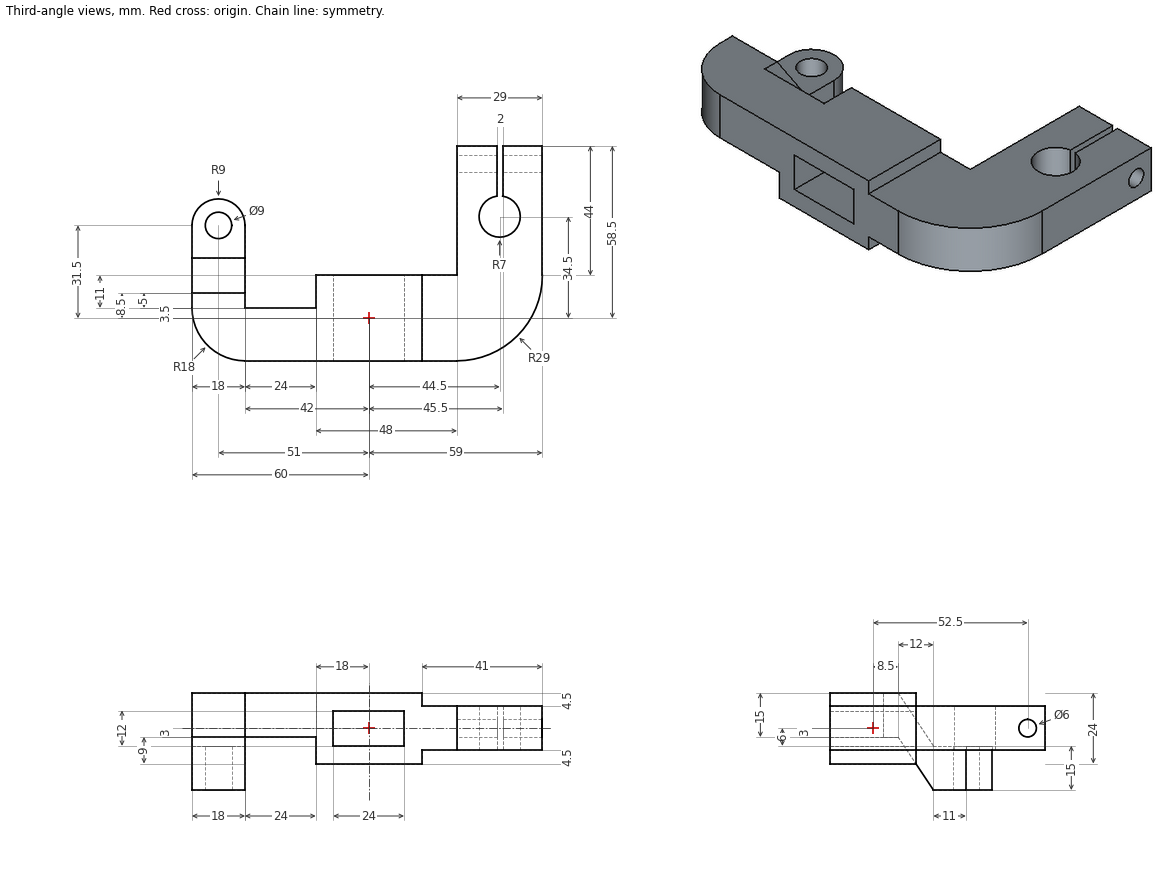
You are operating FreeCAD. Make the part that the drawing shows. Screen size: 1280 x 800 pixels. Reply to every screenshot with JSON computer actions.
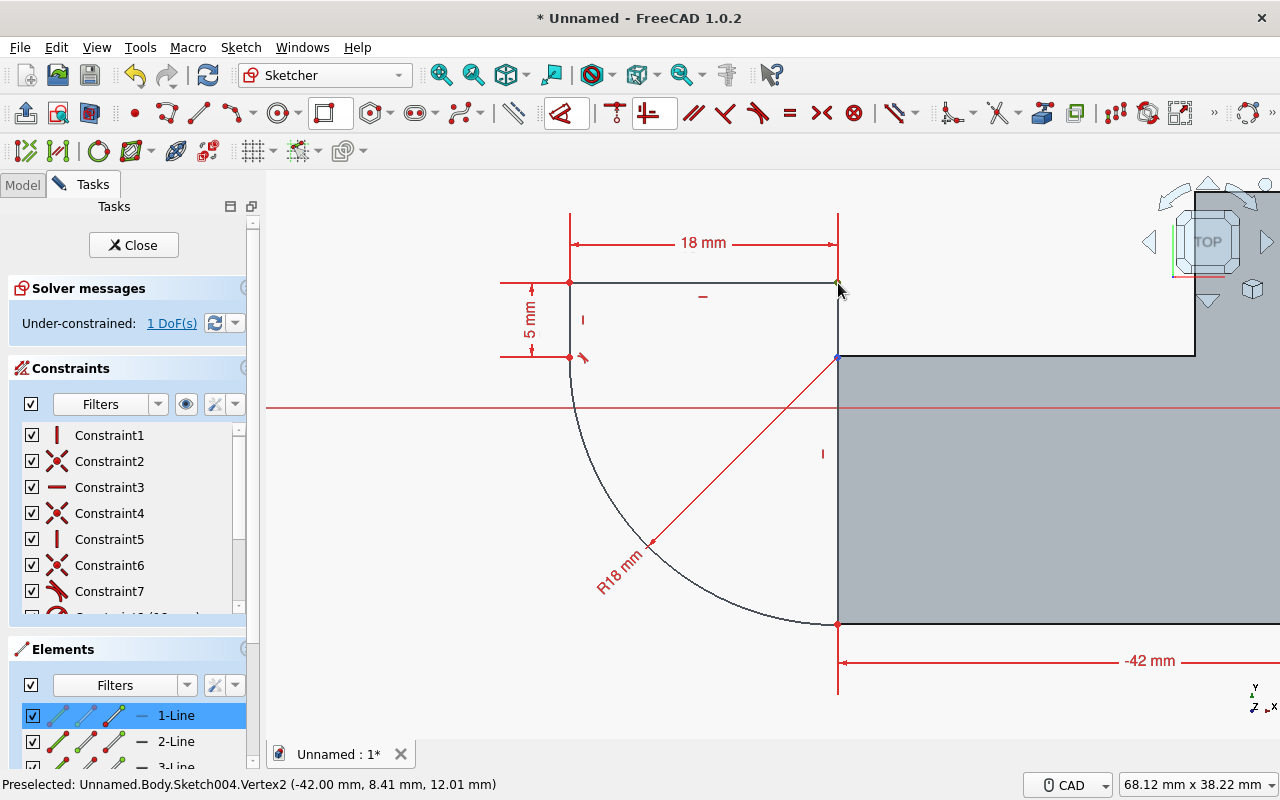
{"action": "key", "text": "i"}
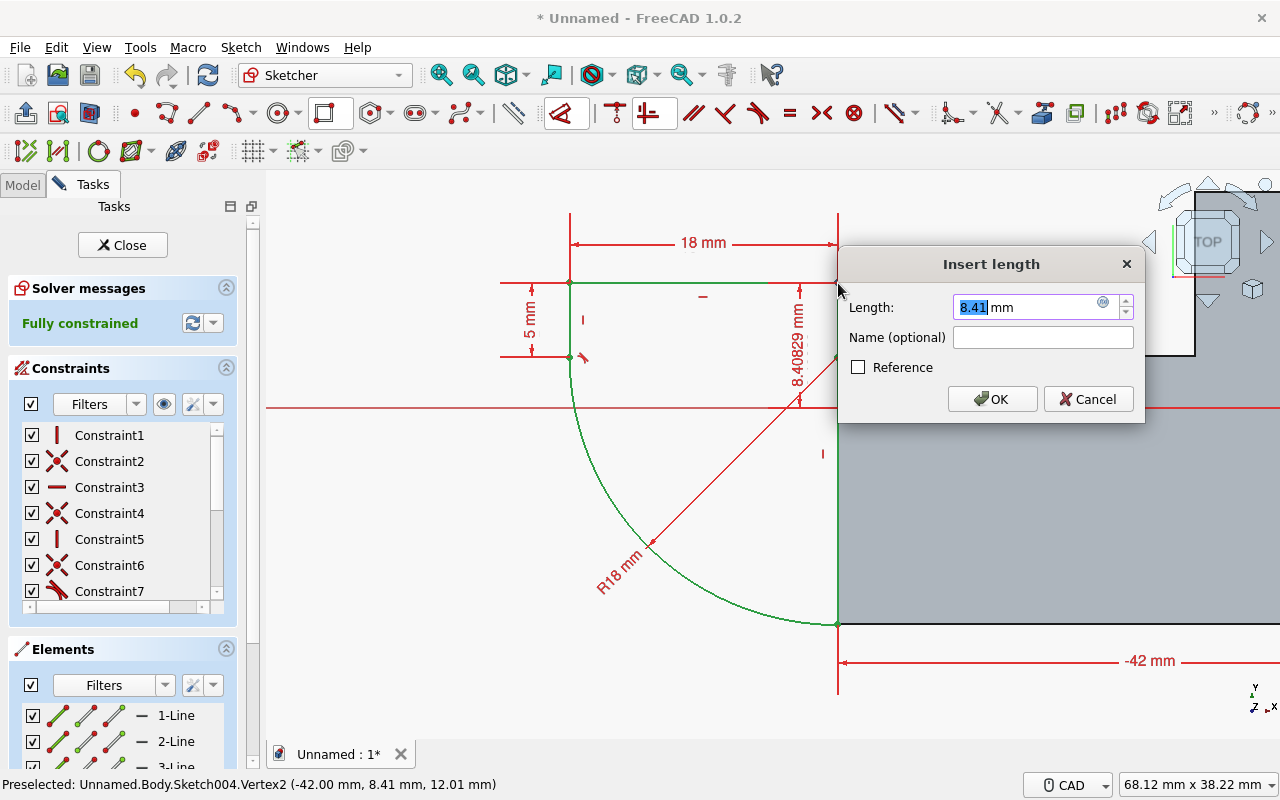
{"action": "type", "text": "8.5"}
{"action": "key", "text": "Return"}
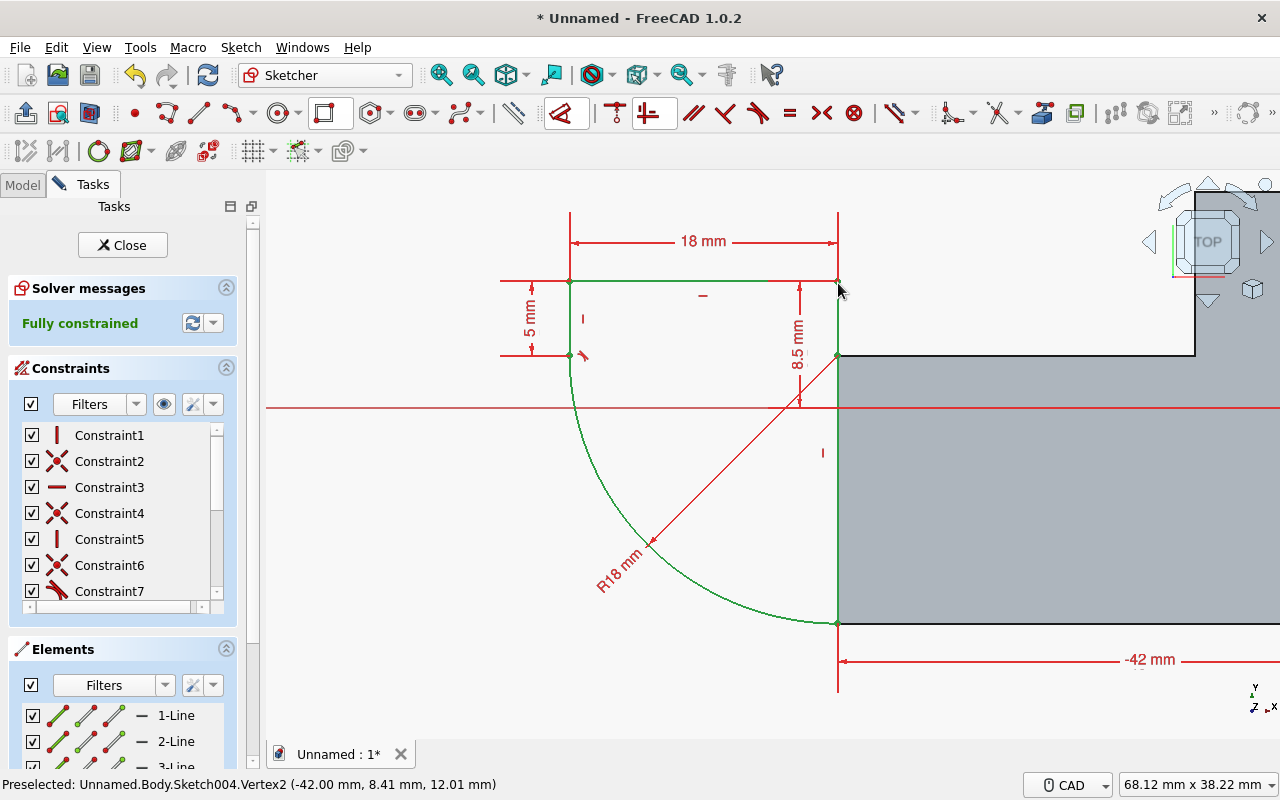
{"action": "left_click", "coordinate": [123, 245]}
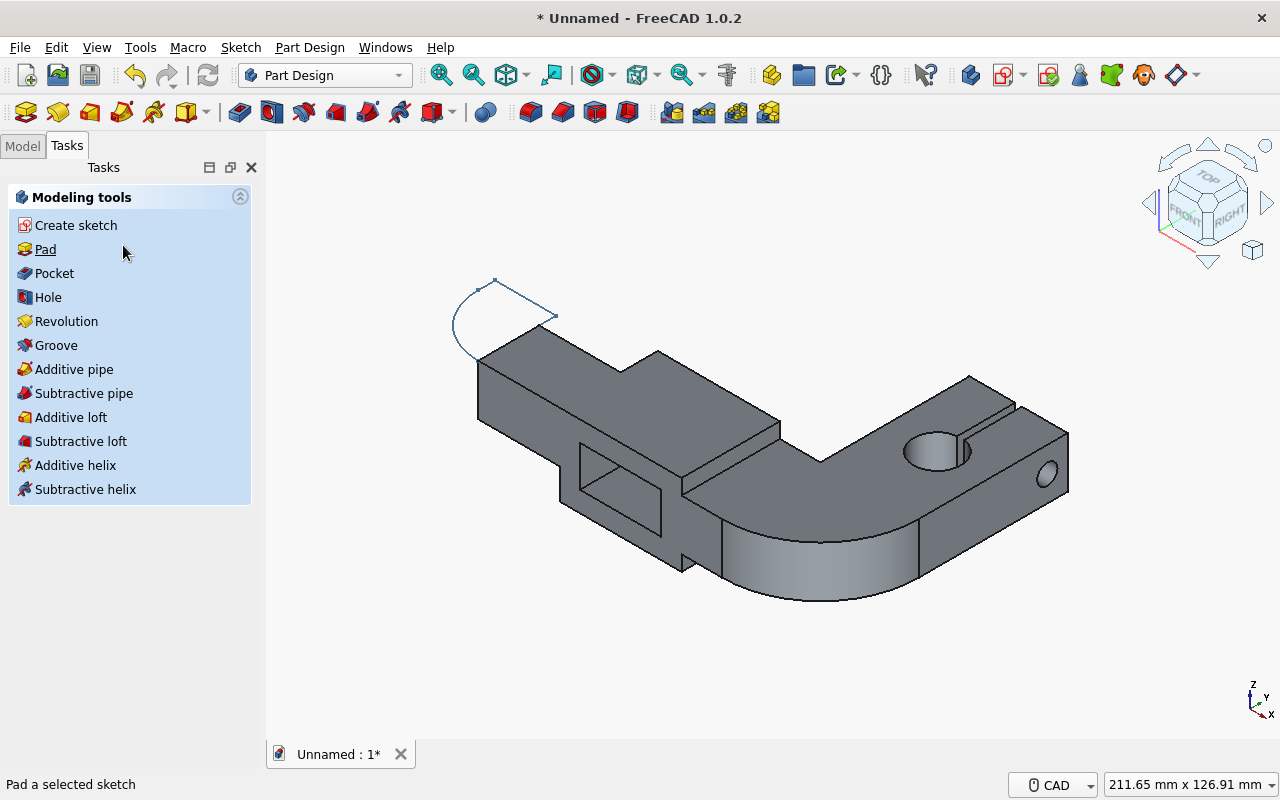
{"action": "left_click", "coordinate": [26, 112]}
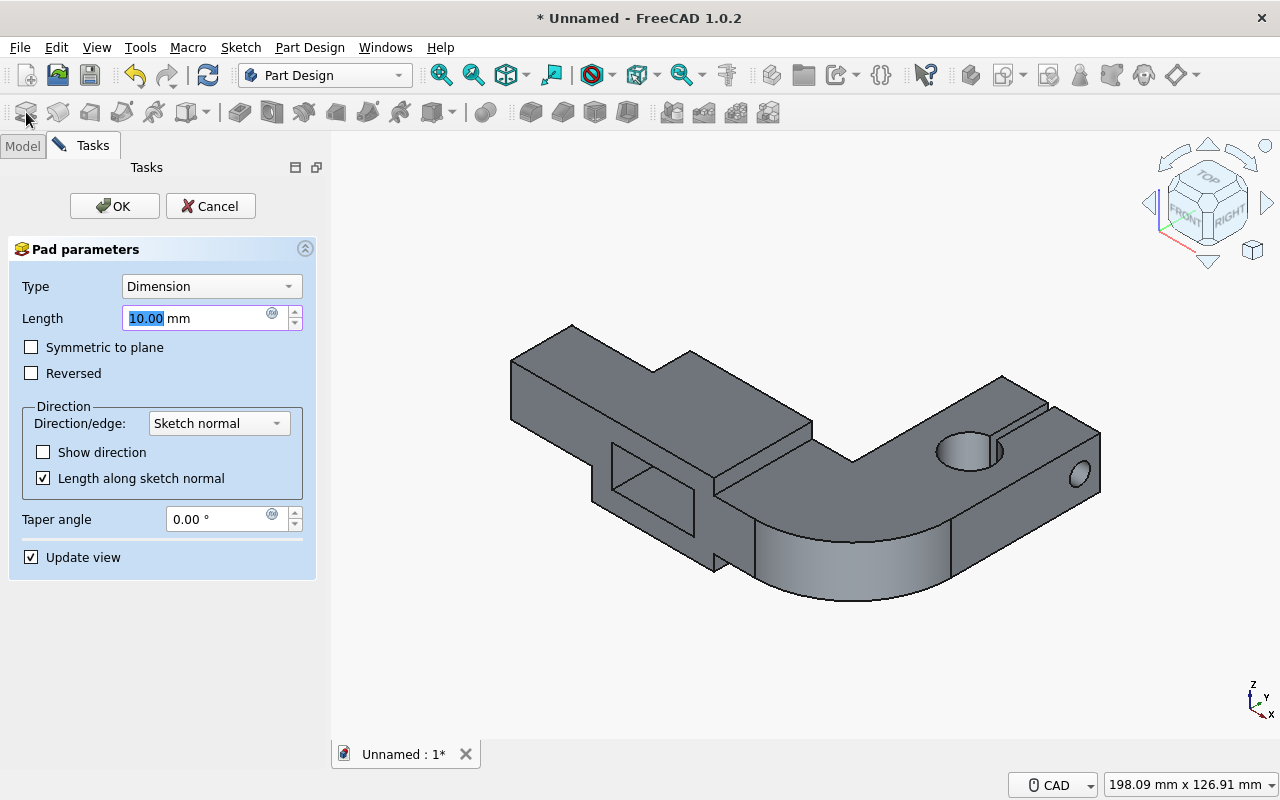
{"action": "type", "text": "15"}
{"action": "key", "text": "Tab"}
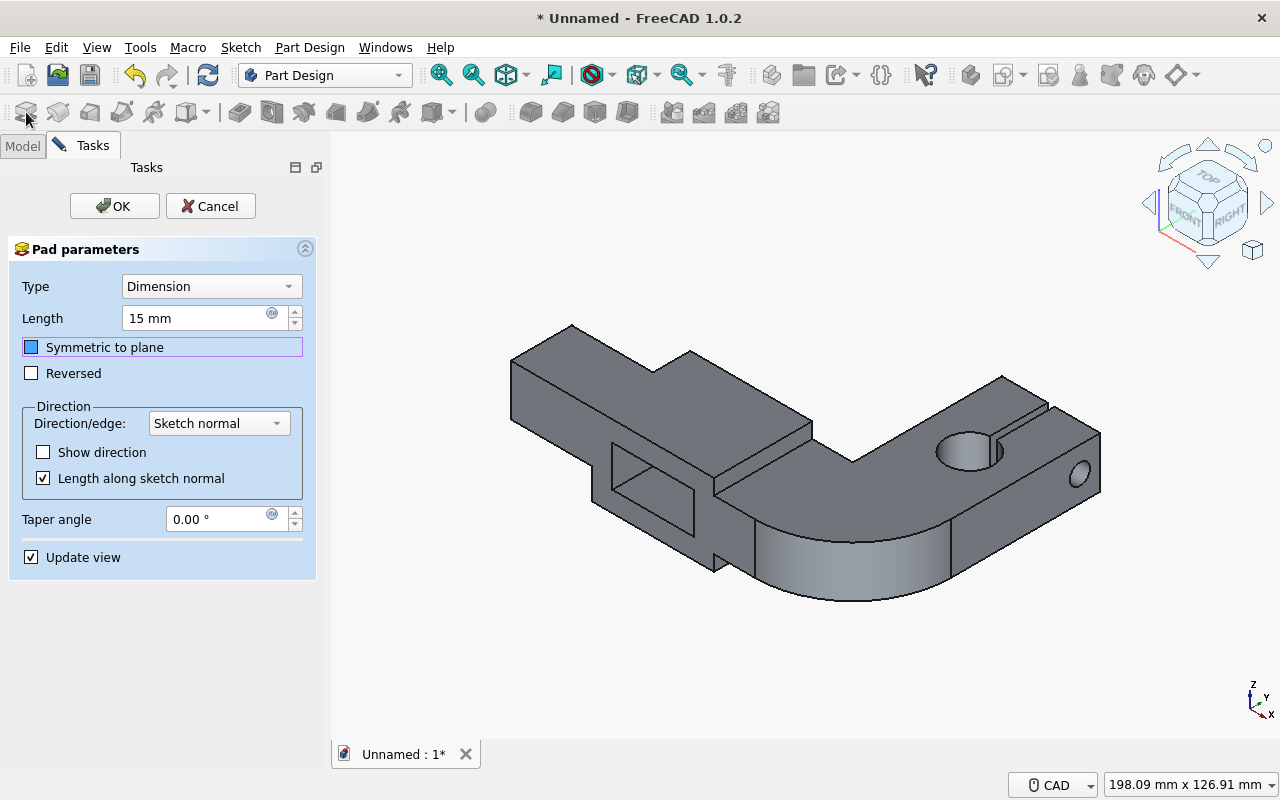
{"action": "left_click", "coordinate": [30, 373]}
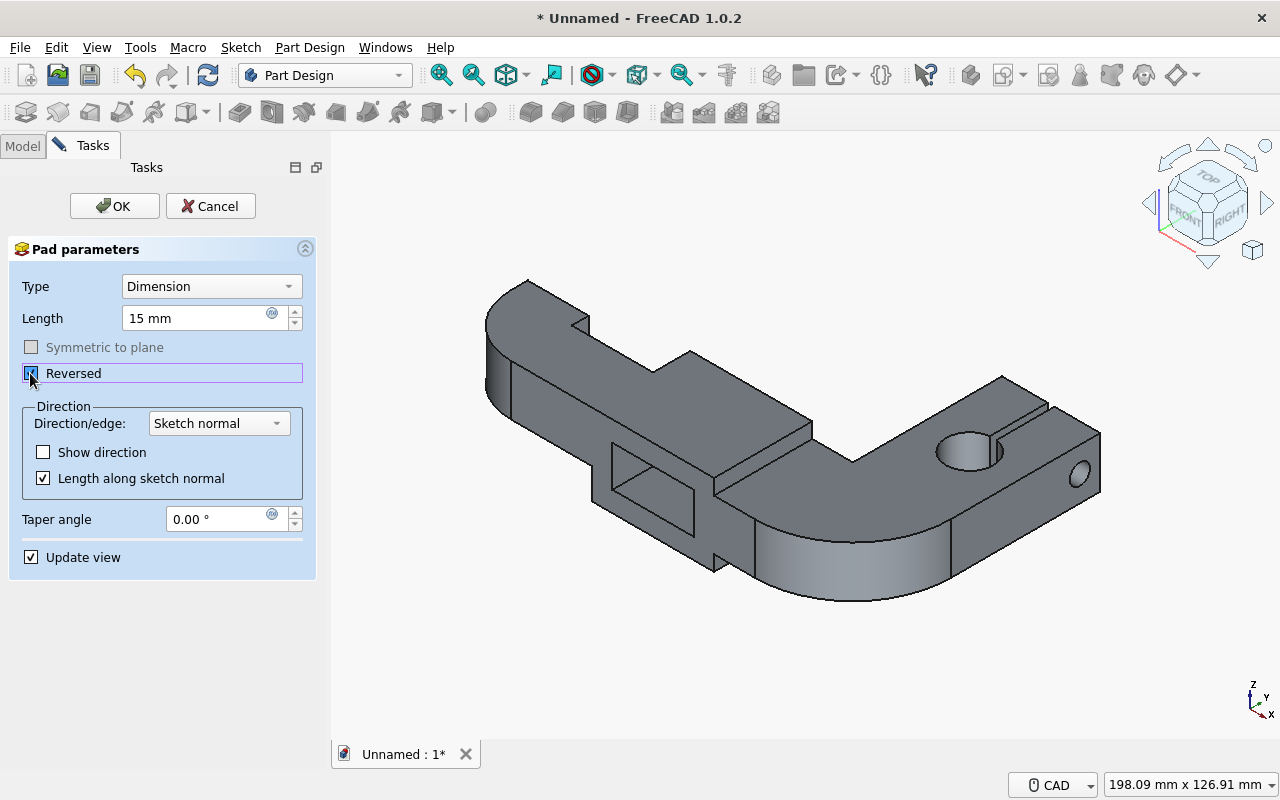
{"action": "left_click", "coordinate": [115, 206]}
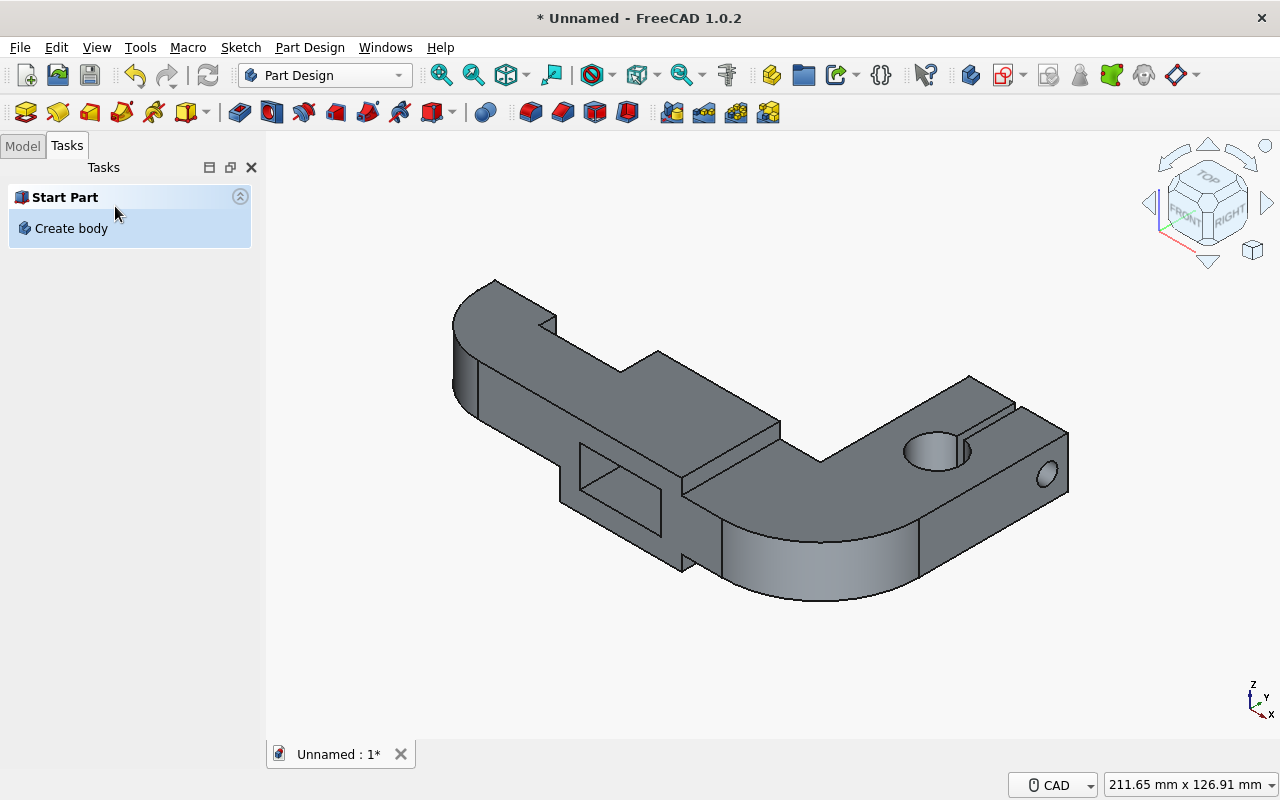
{"action": "key", "text": "6"}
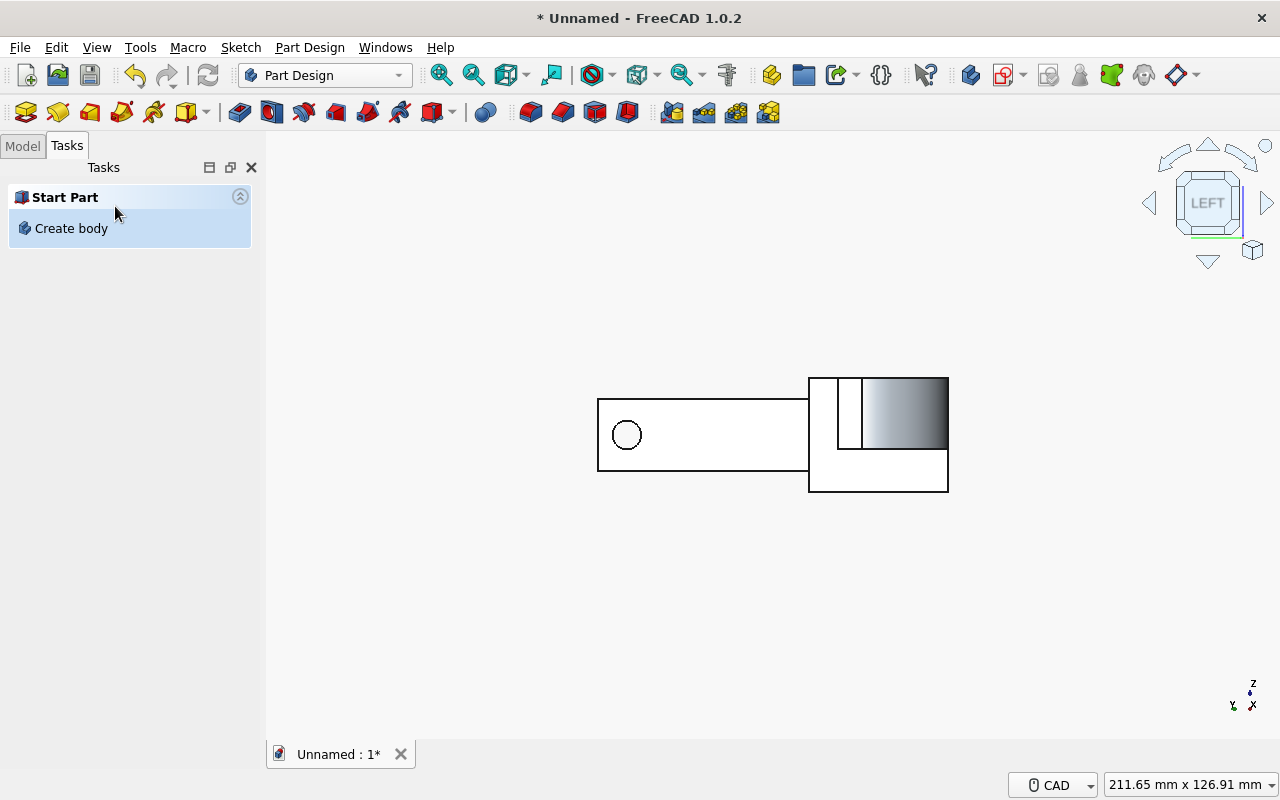
{"action": "left_click", "coordinate": [442, 76]}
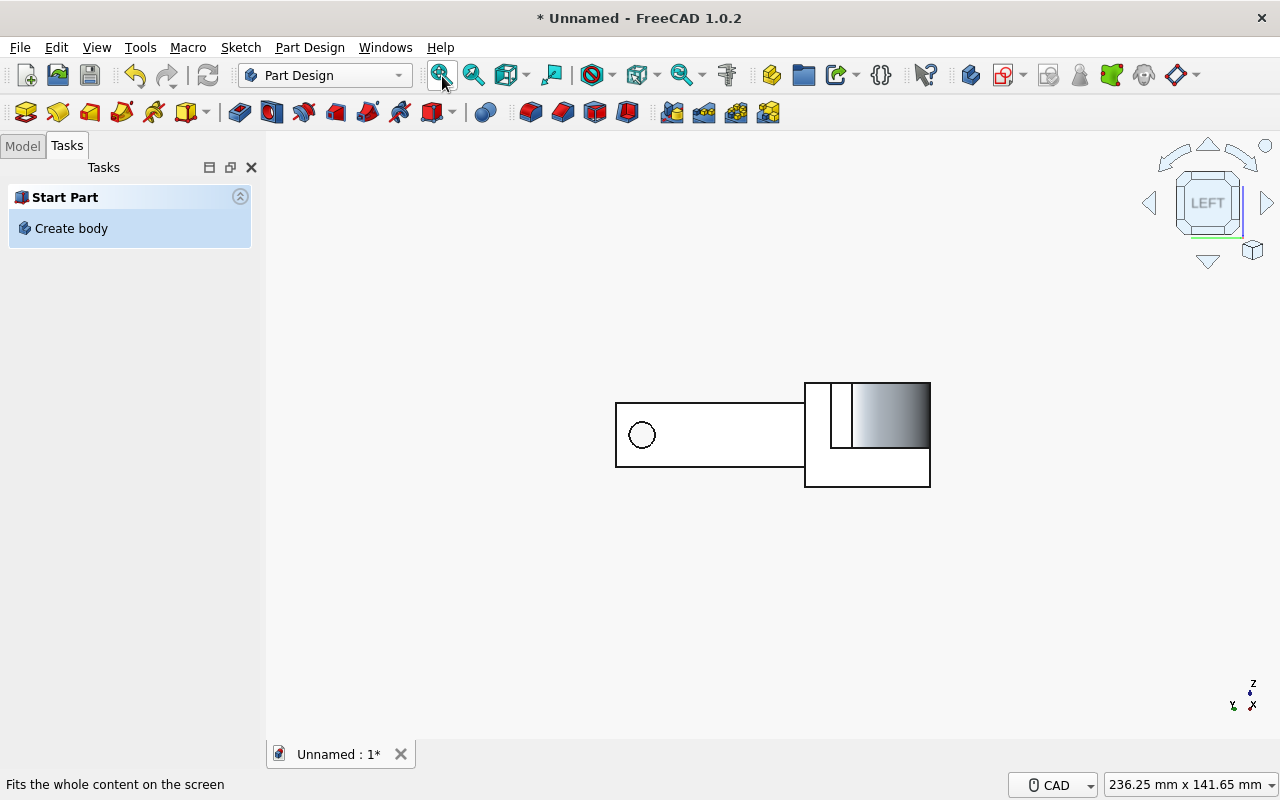
{"action": "left_click", "coordinate": [842, 396]}